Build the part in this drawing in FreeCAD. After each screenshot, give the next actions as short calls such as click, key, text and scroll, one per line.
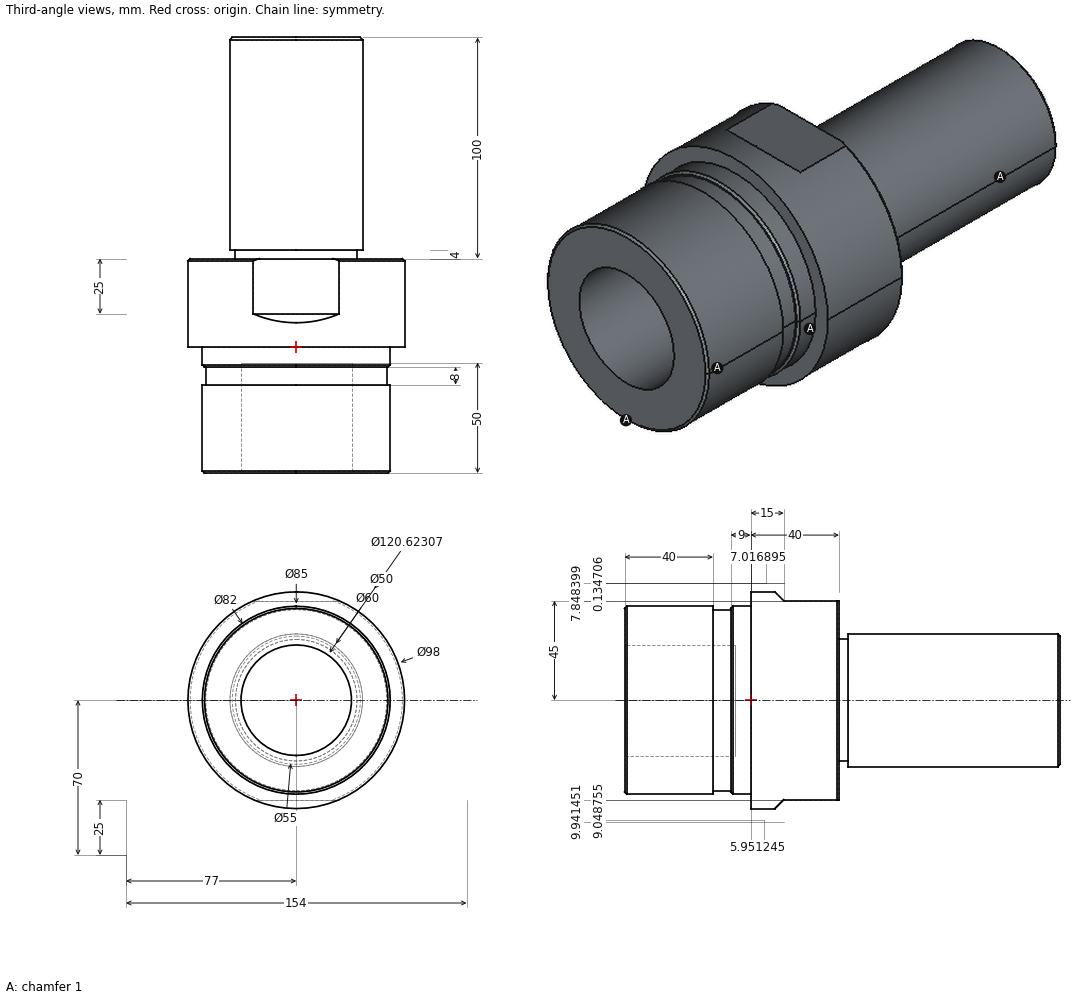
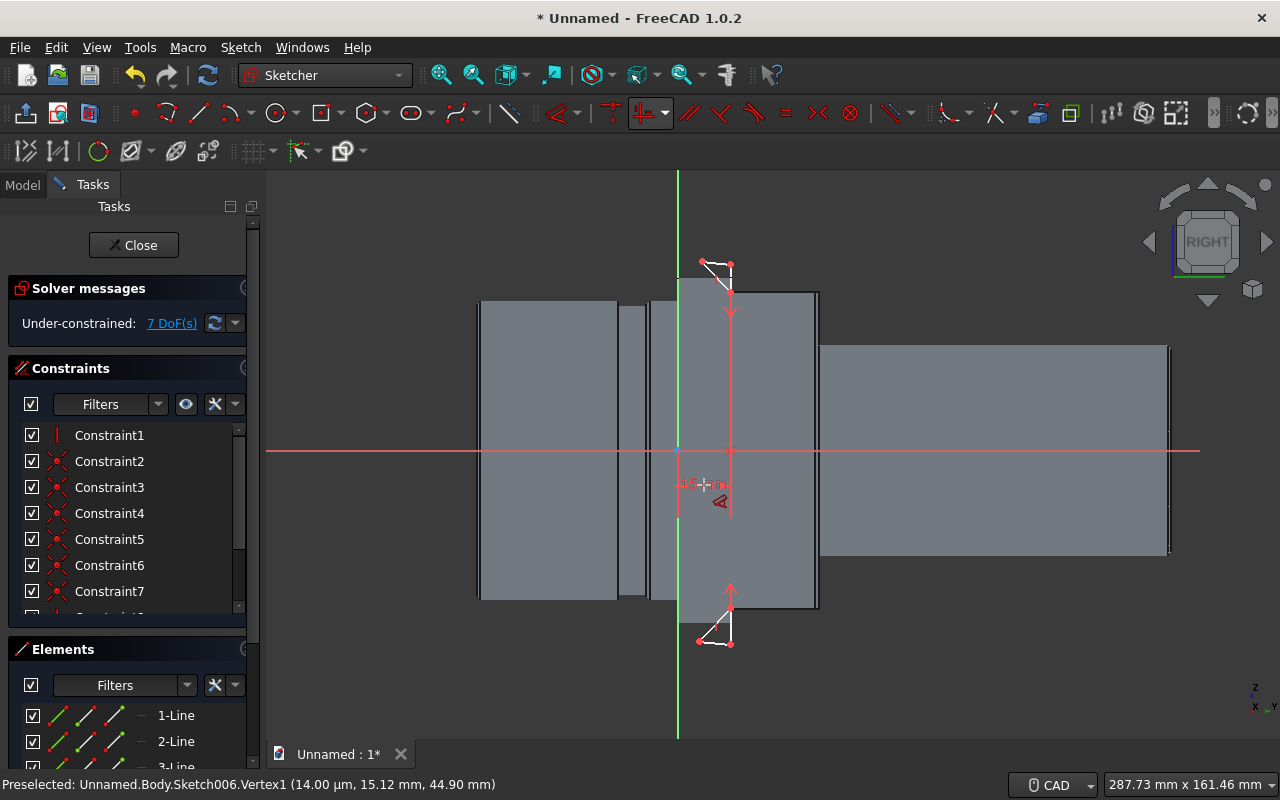
click(731, 292)
click(765, 371)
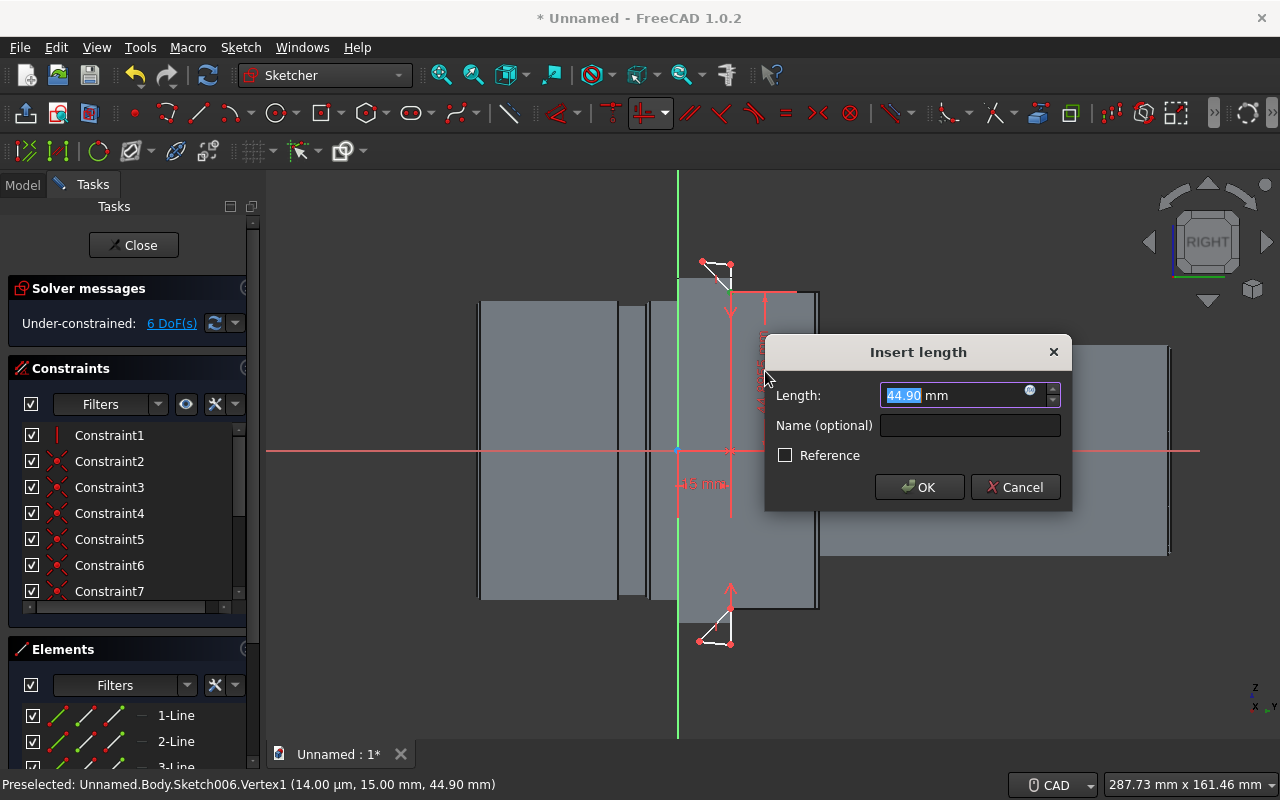
text(45)
key(Return)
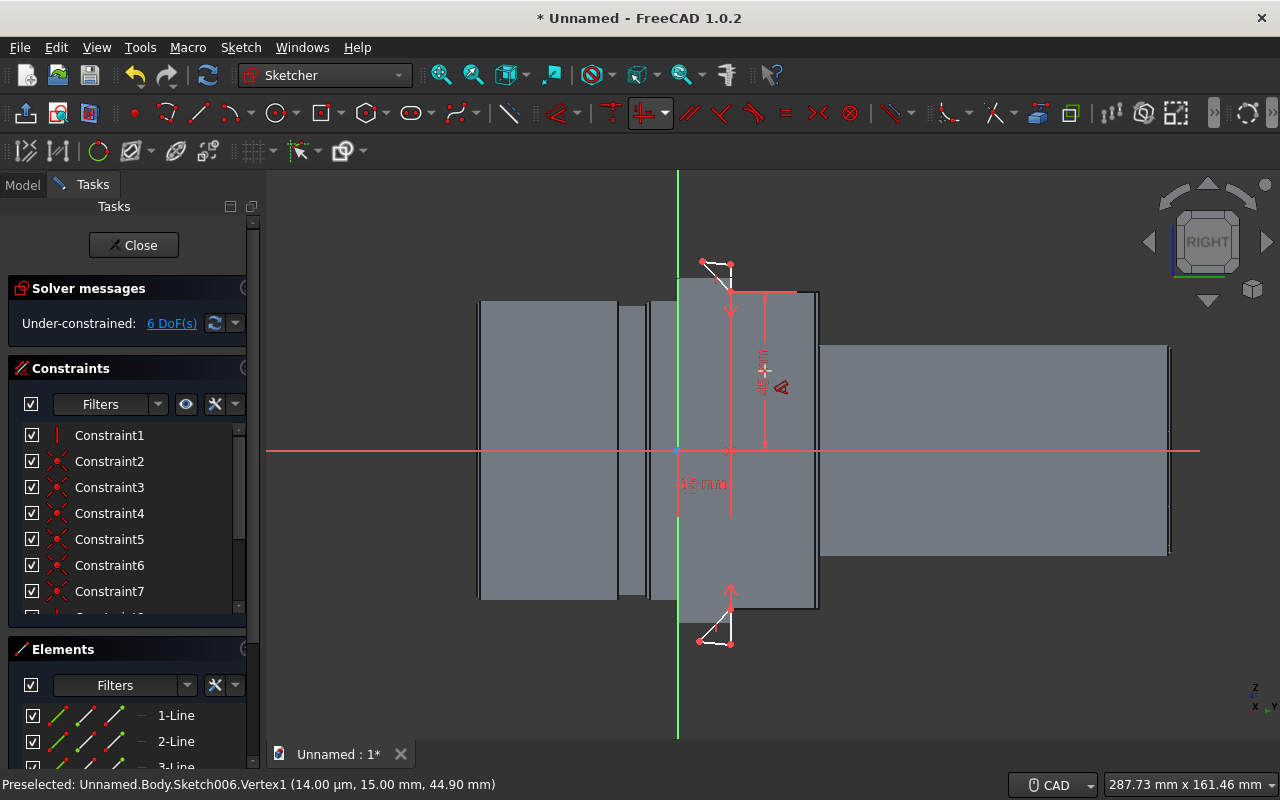
scroll(731, 276, up, 2)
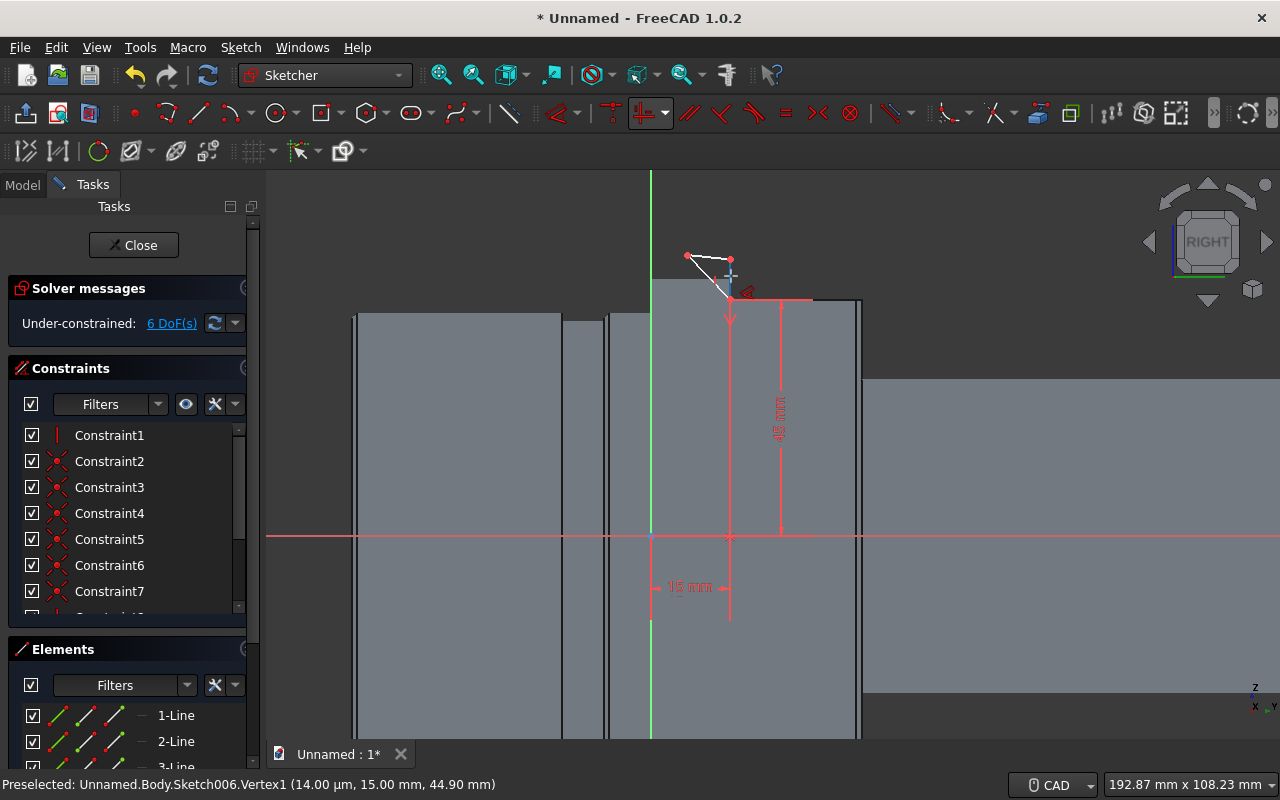
click(730, 276)
click(764, 280)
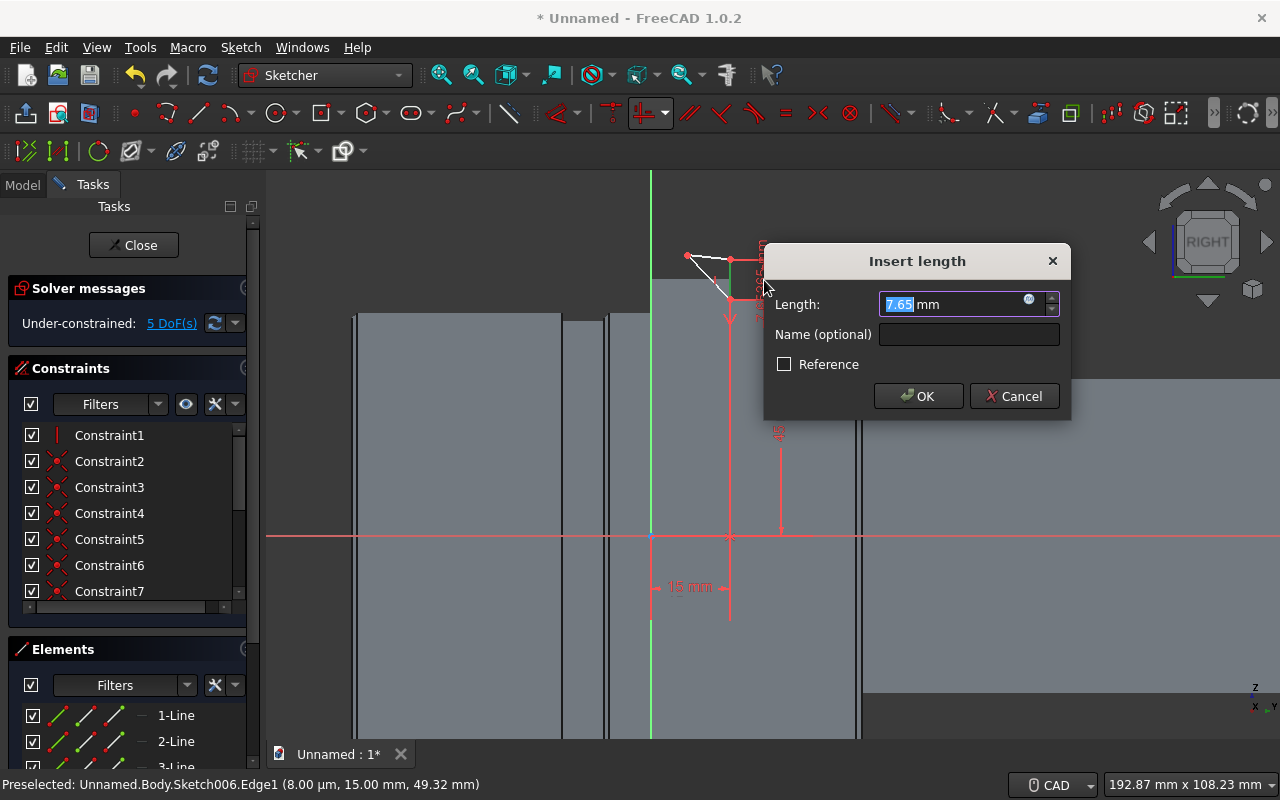
text(7.848399)
key(Return)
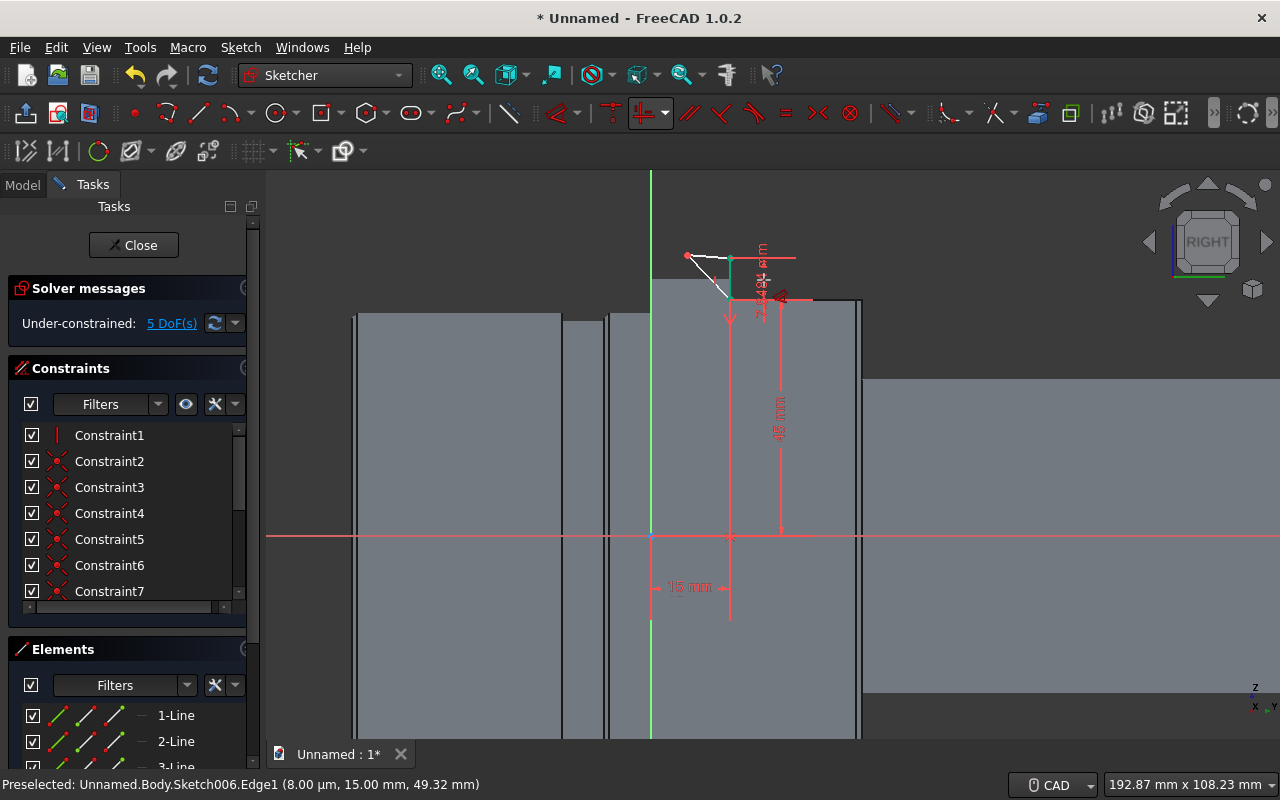
scroll(733, 278, down, 2)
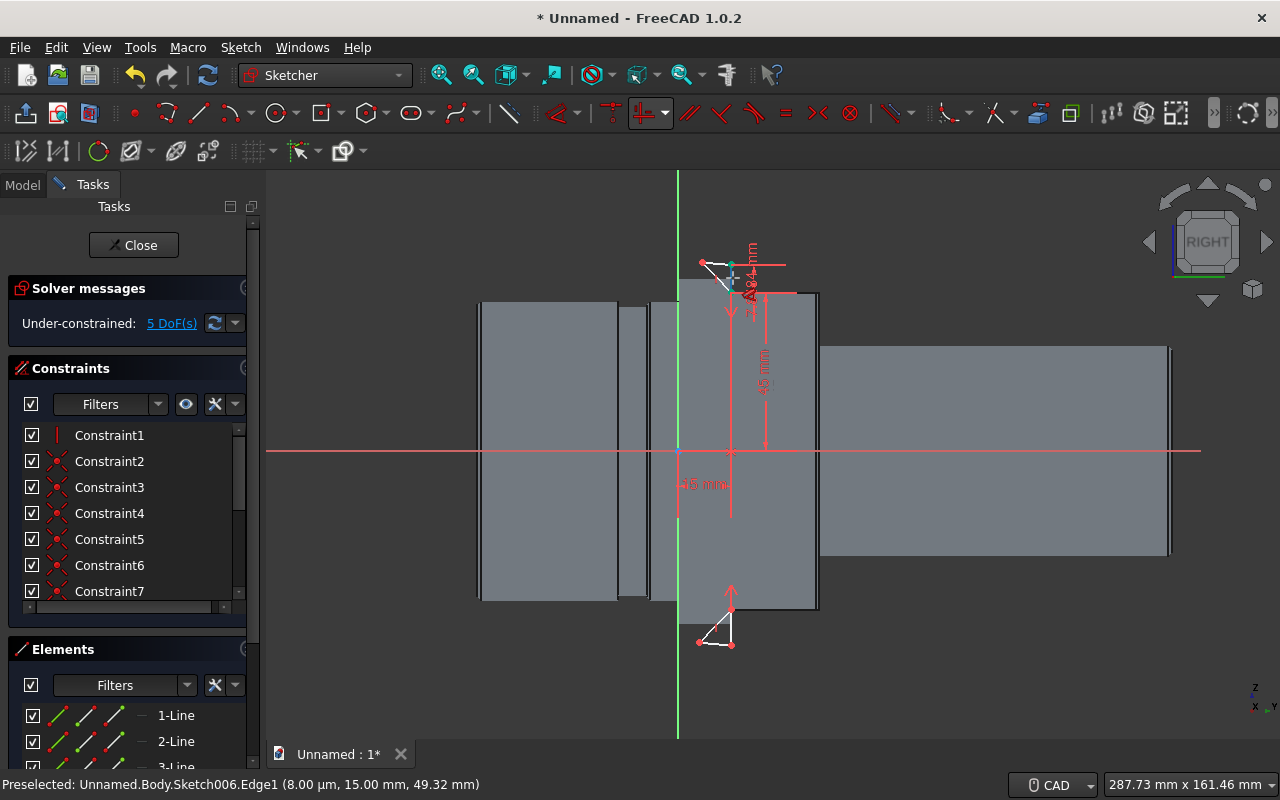
scroll(731, 635, up, 2)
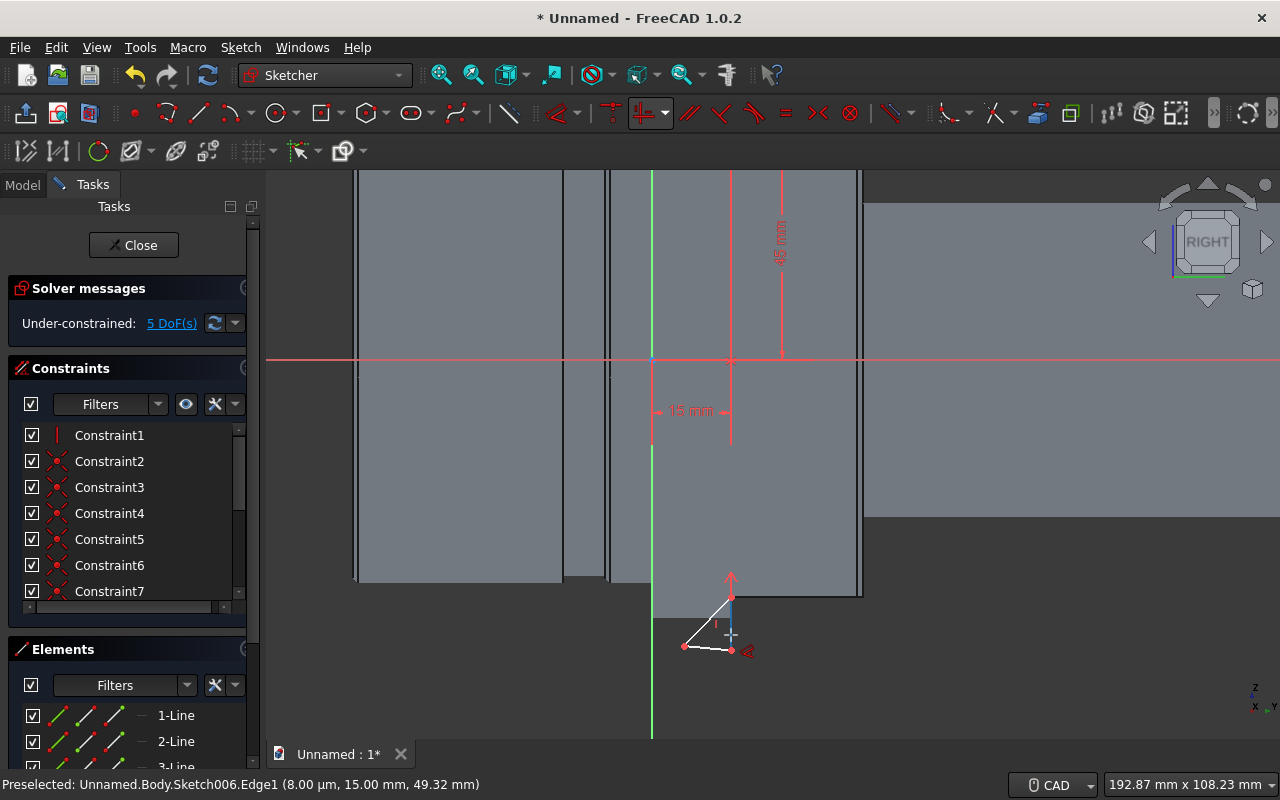
click(731, 634)
click(765, 624)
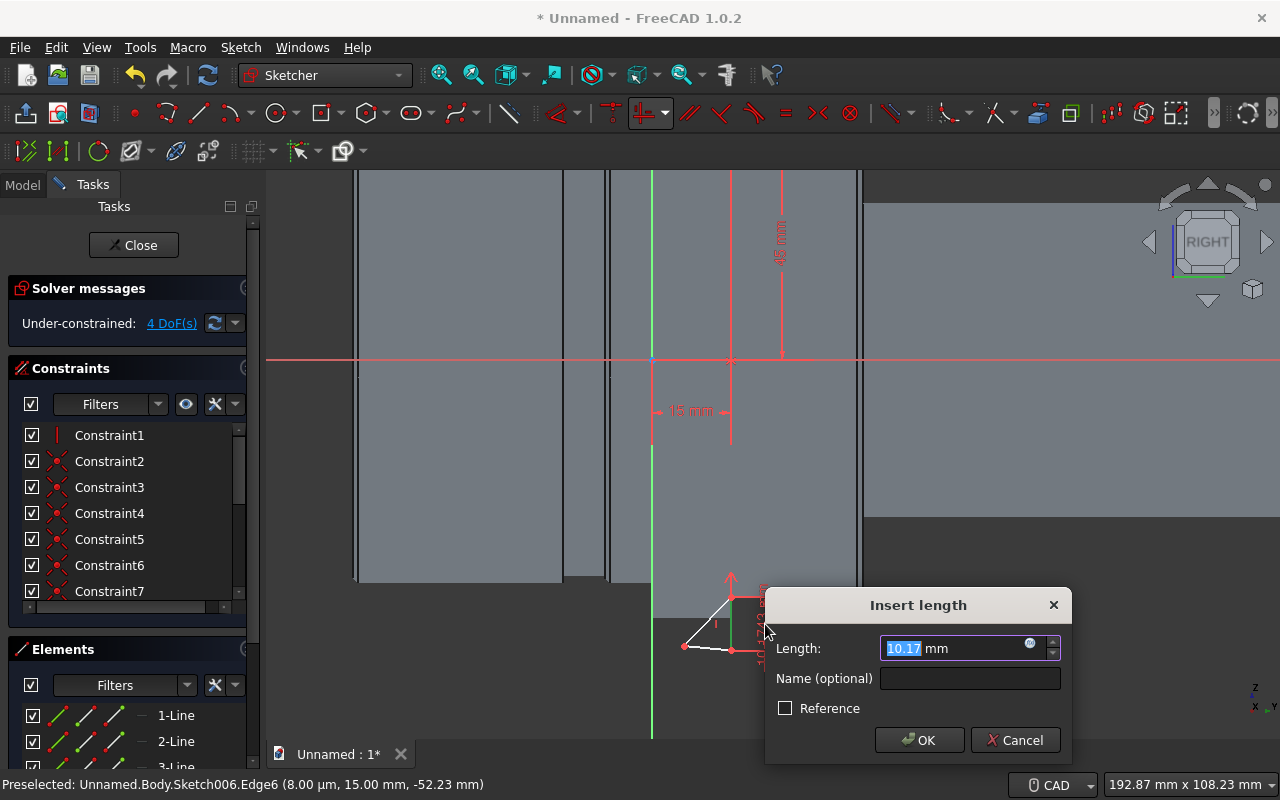
text(9.941451)
key(Return)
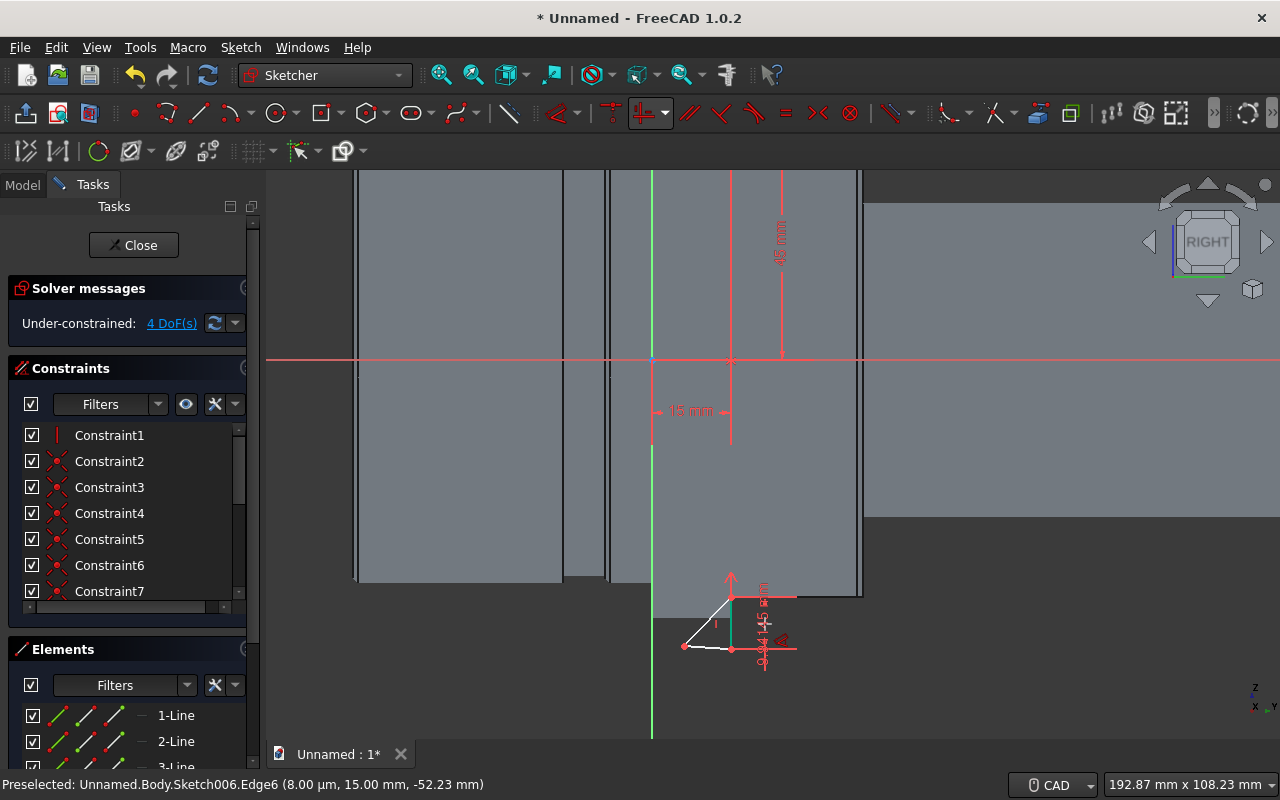
scroll(731, 635, down, 2)